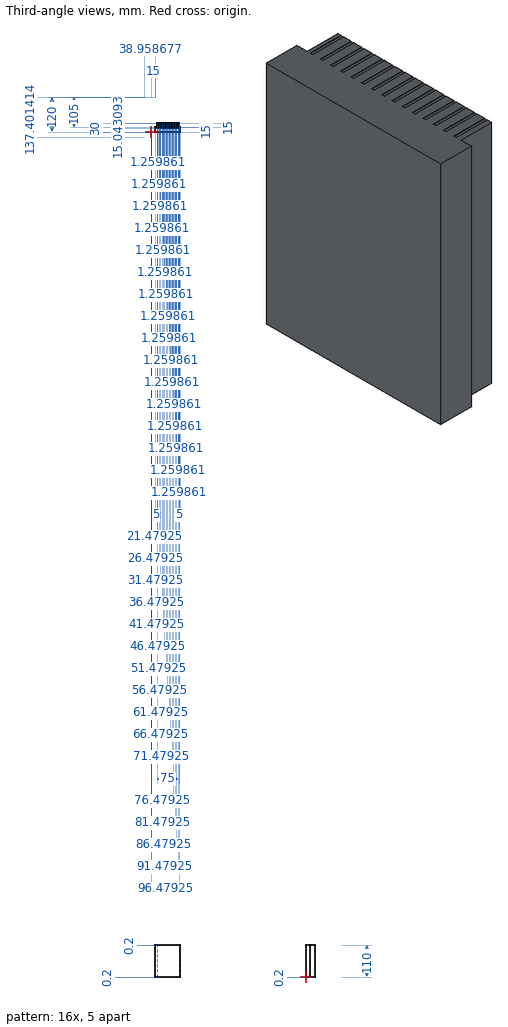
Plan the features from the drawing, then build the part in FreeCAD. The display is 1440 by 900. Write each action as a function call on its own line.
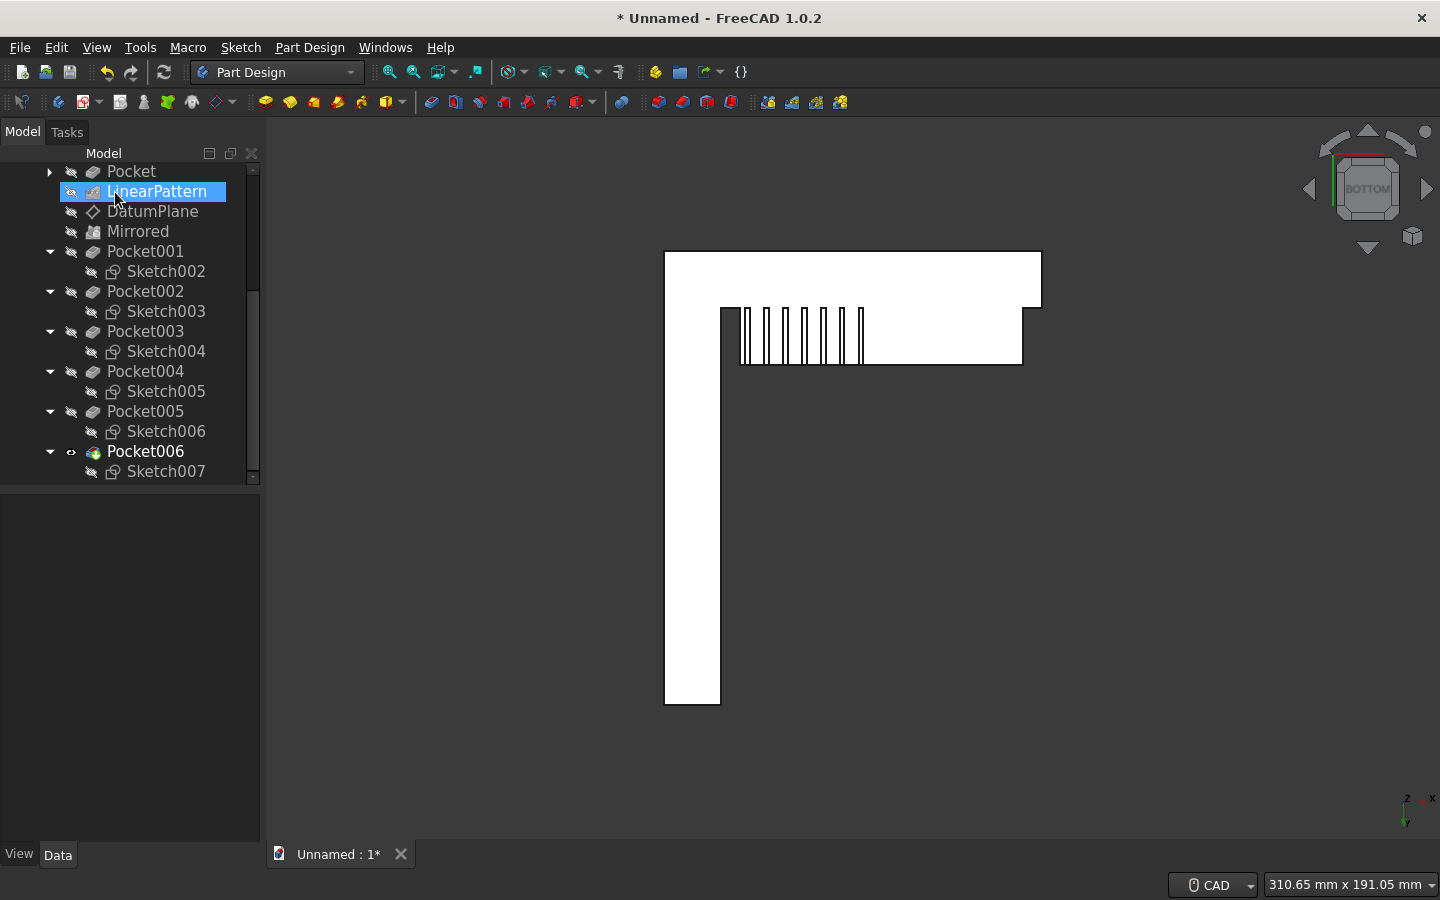
click(961, 283)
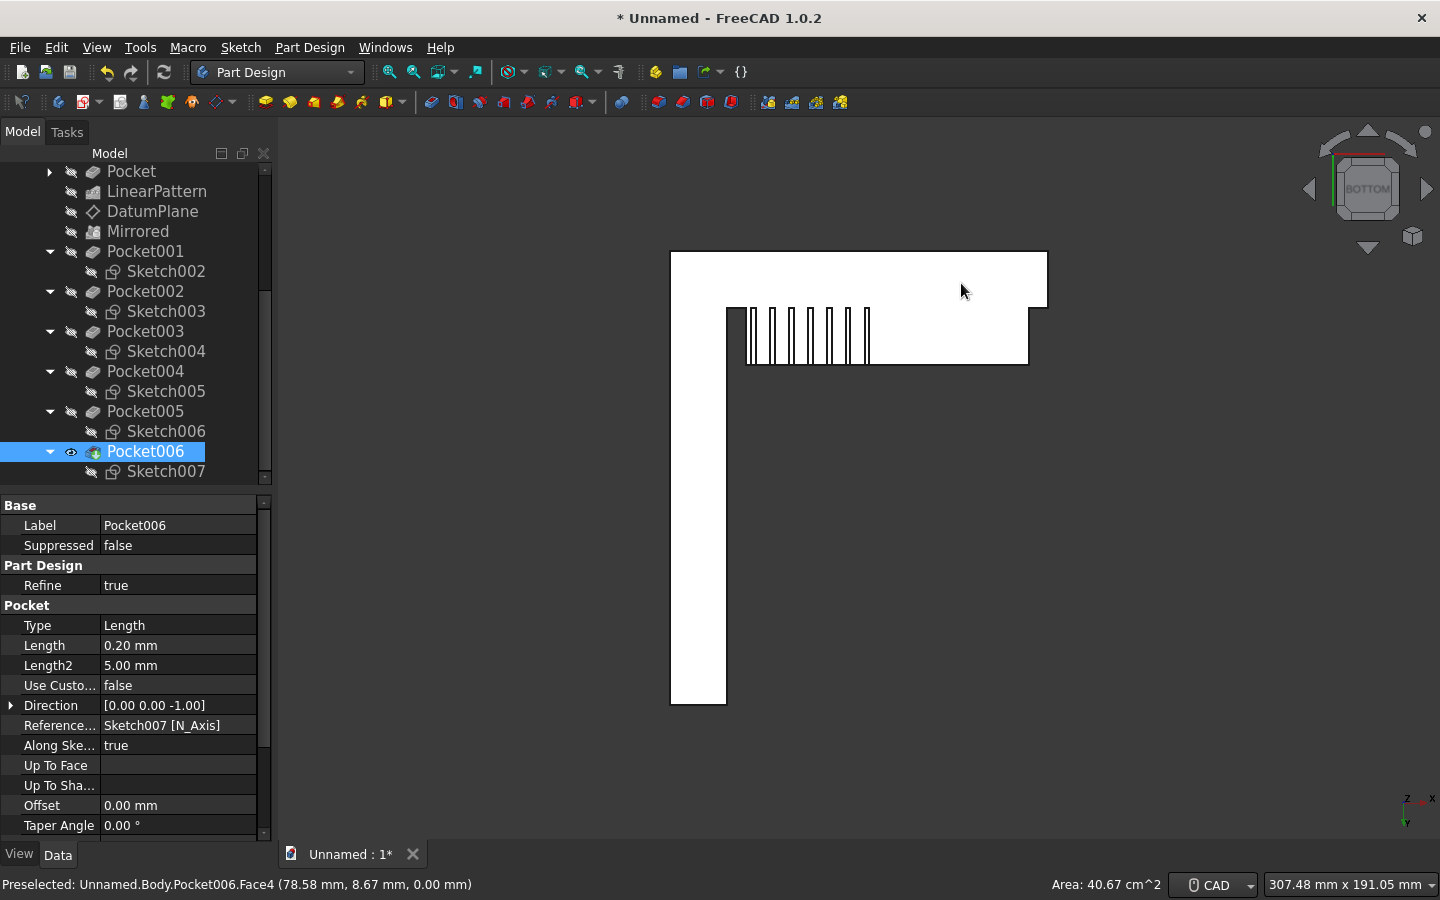
click(84, 102)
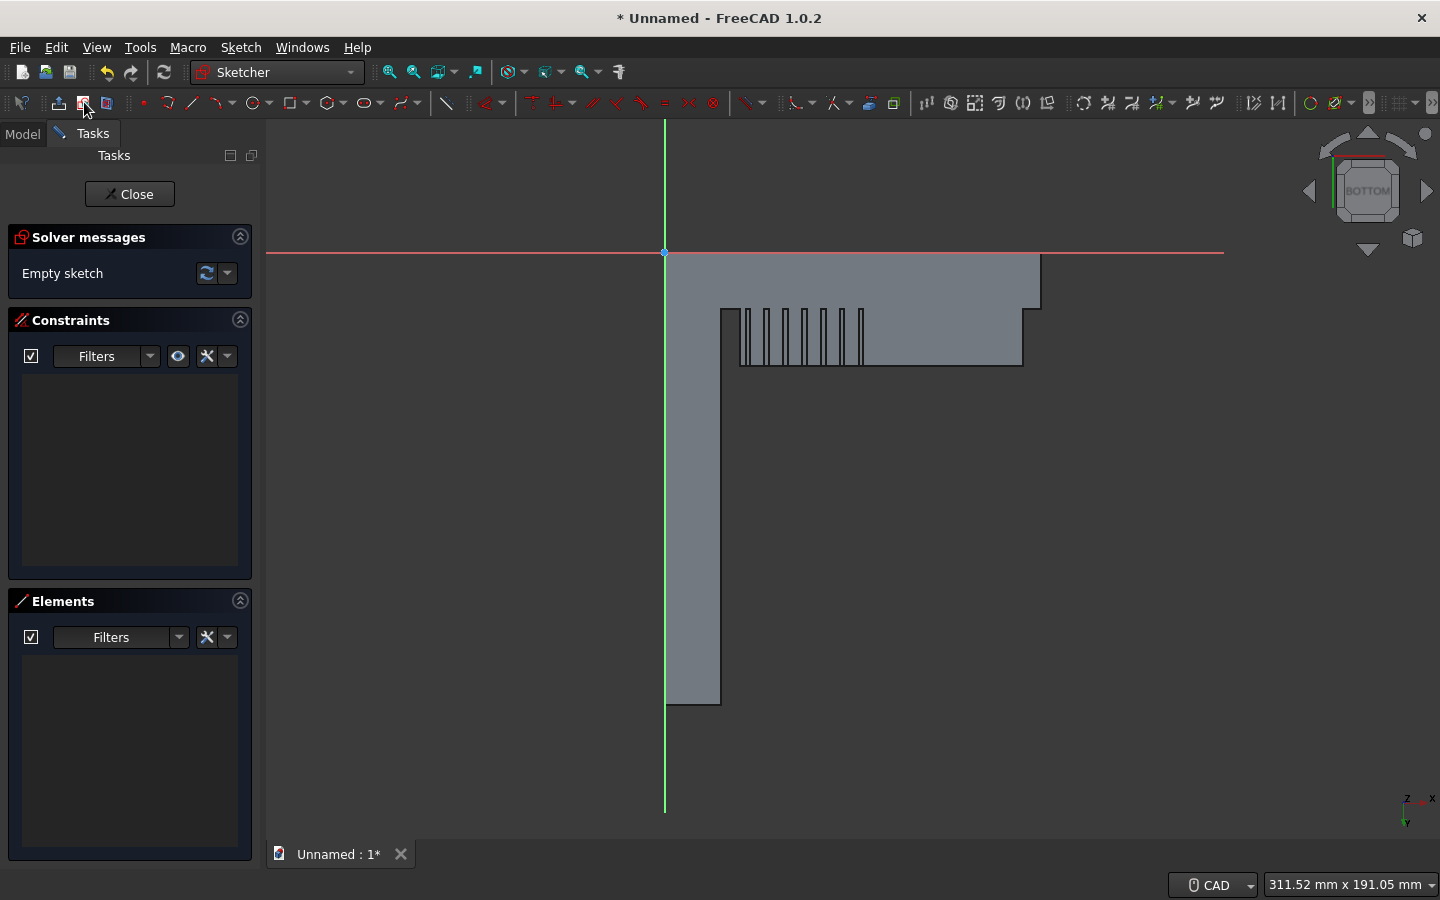
scroll(892, 320, up, 11)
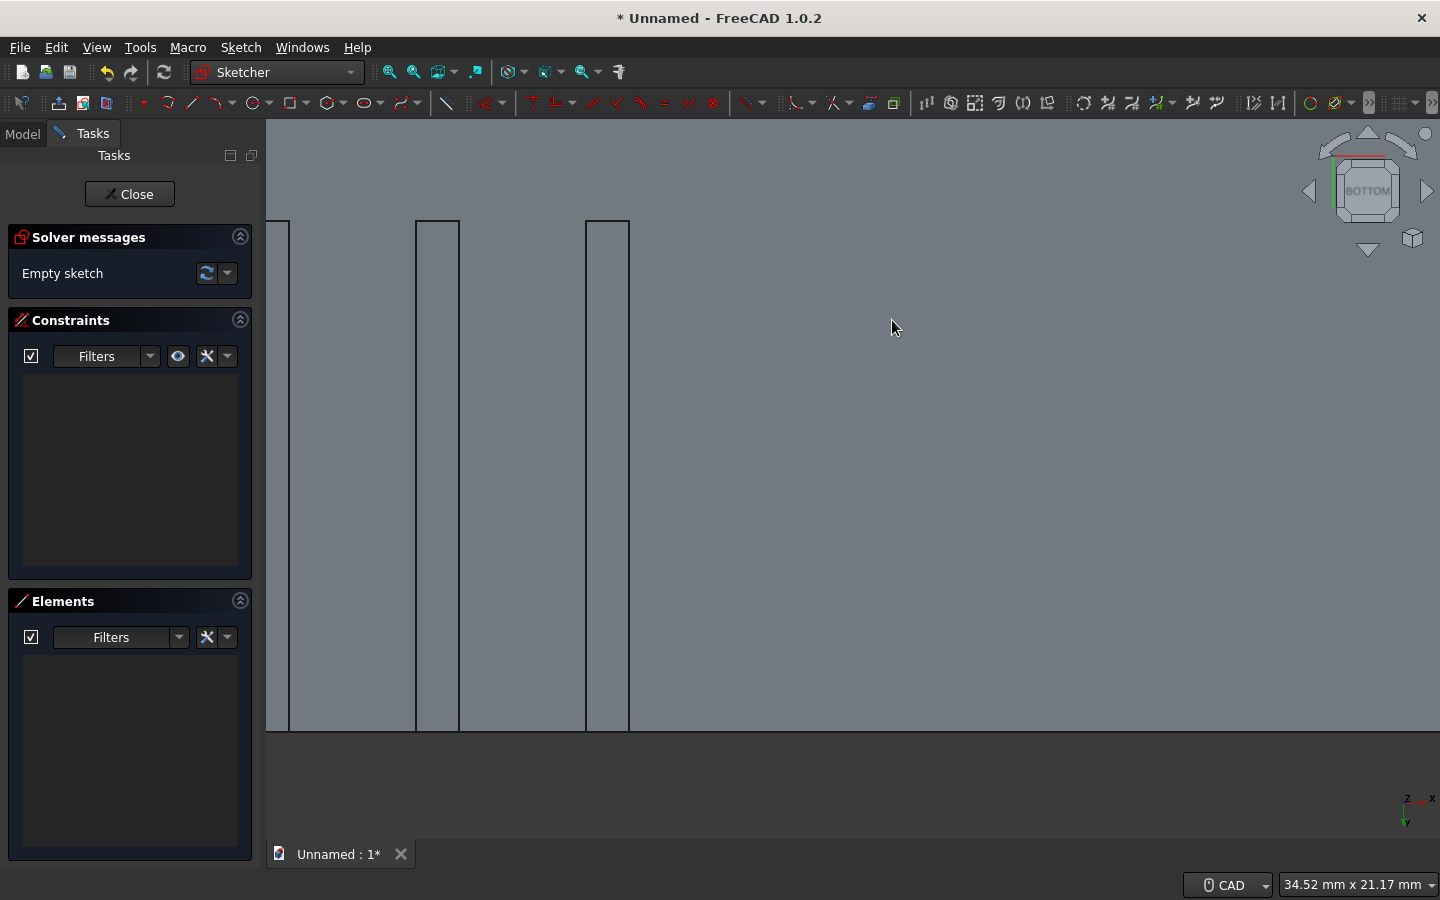
click(290, 104)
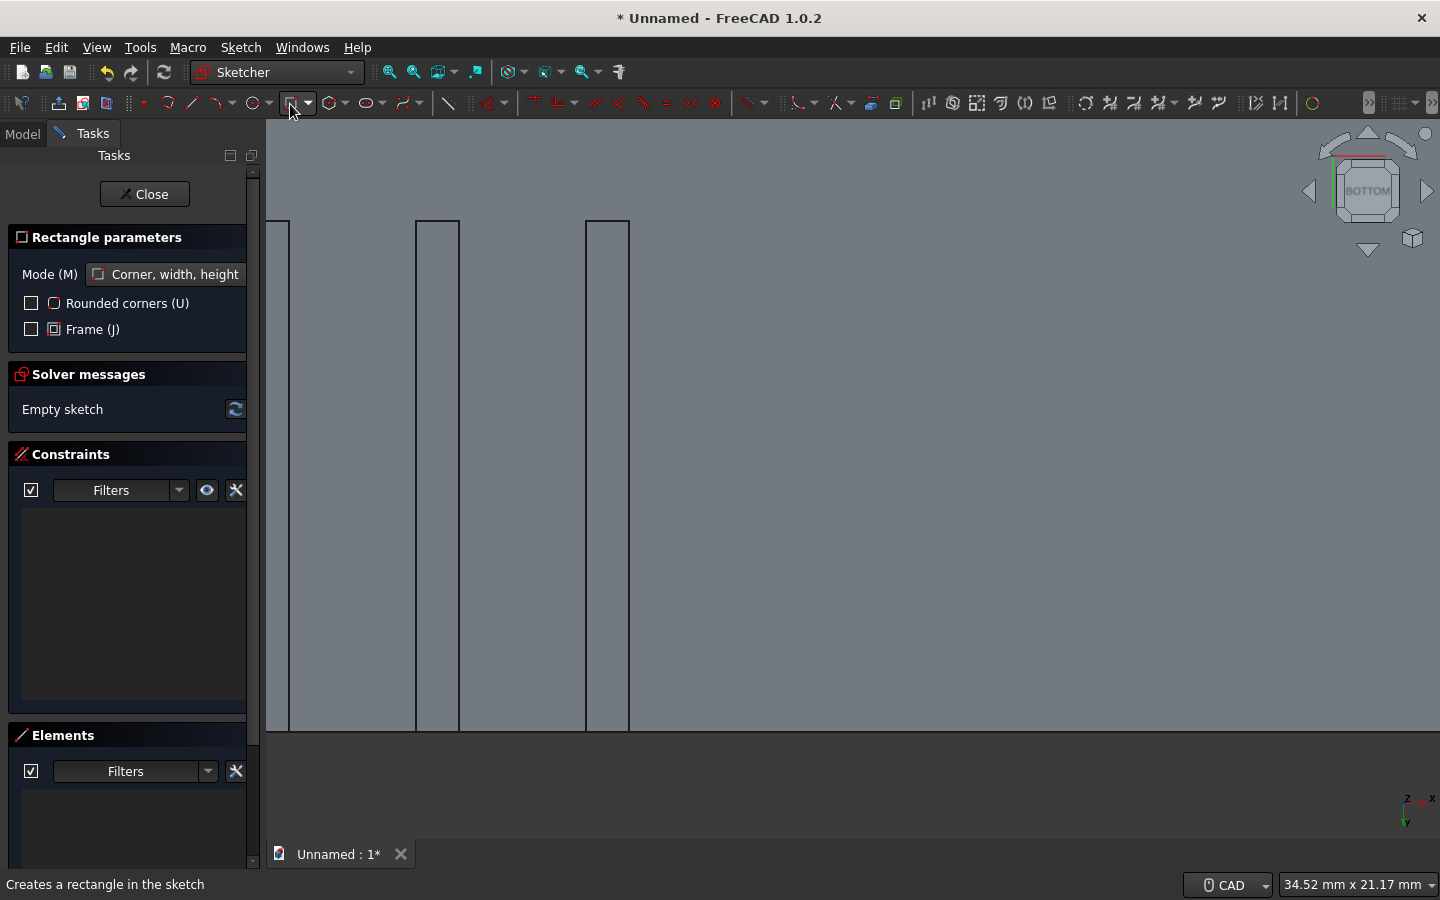
click(756, 221)
click(799, 732)
key(Escape)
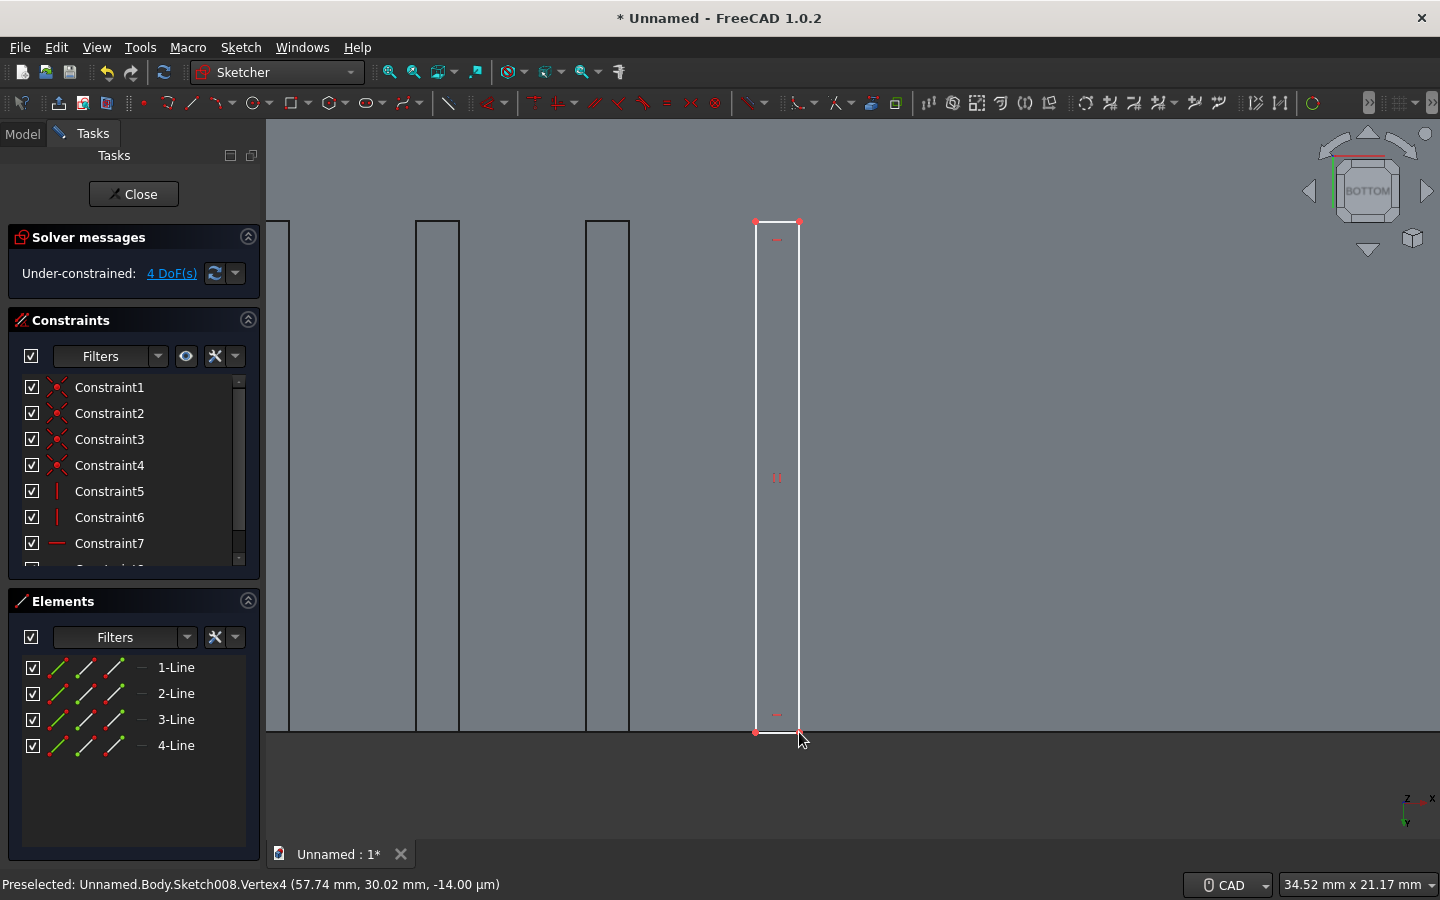
click(488, 104)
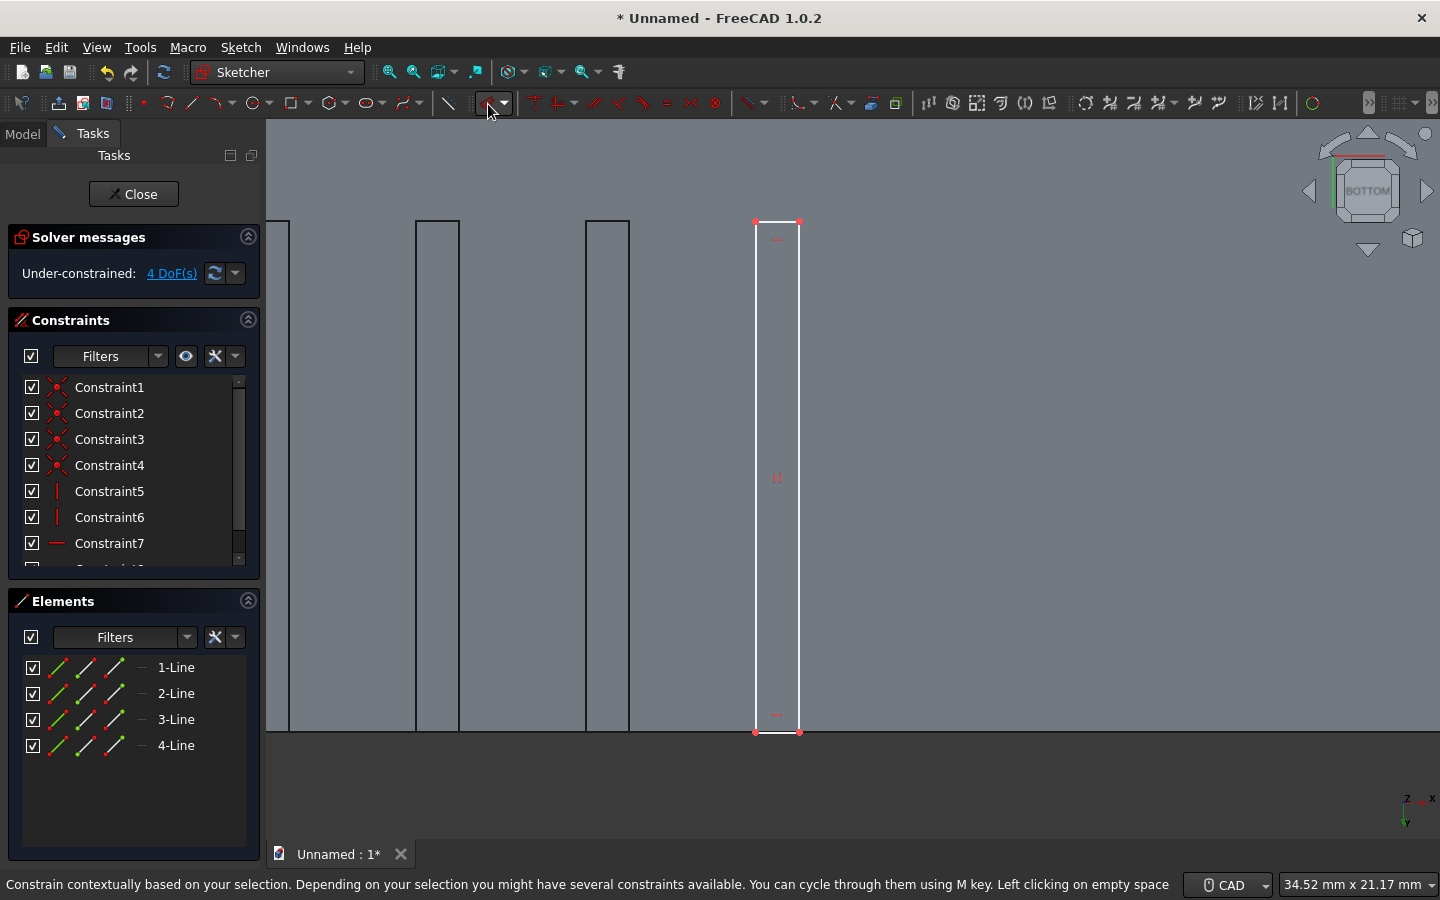
click(756, 733)
click(814, 440)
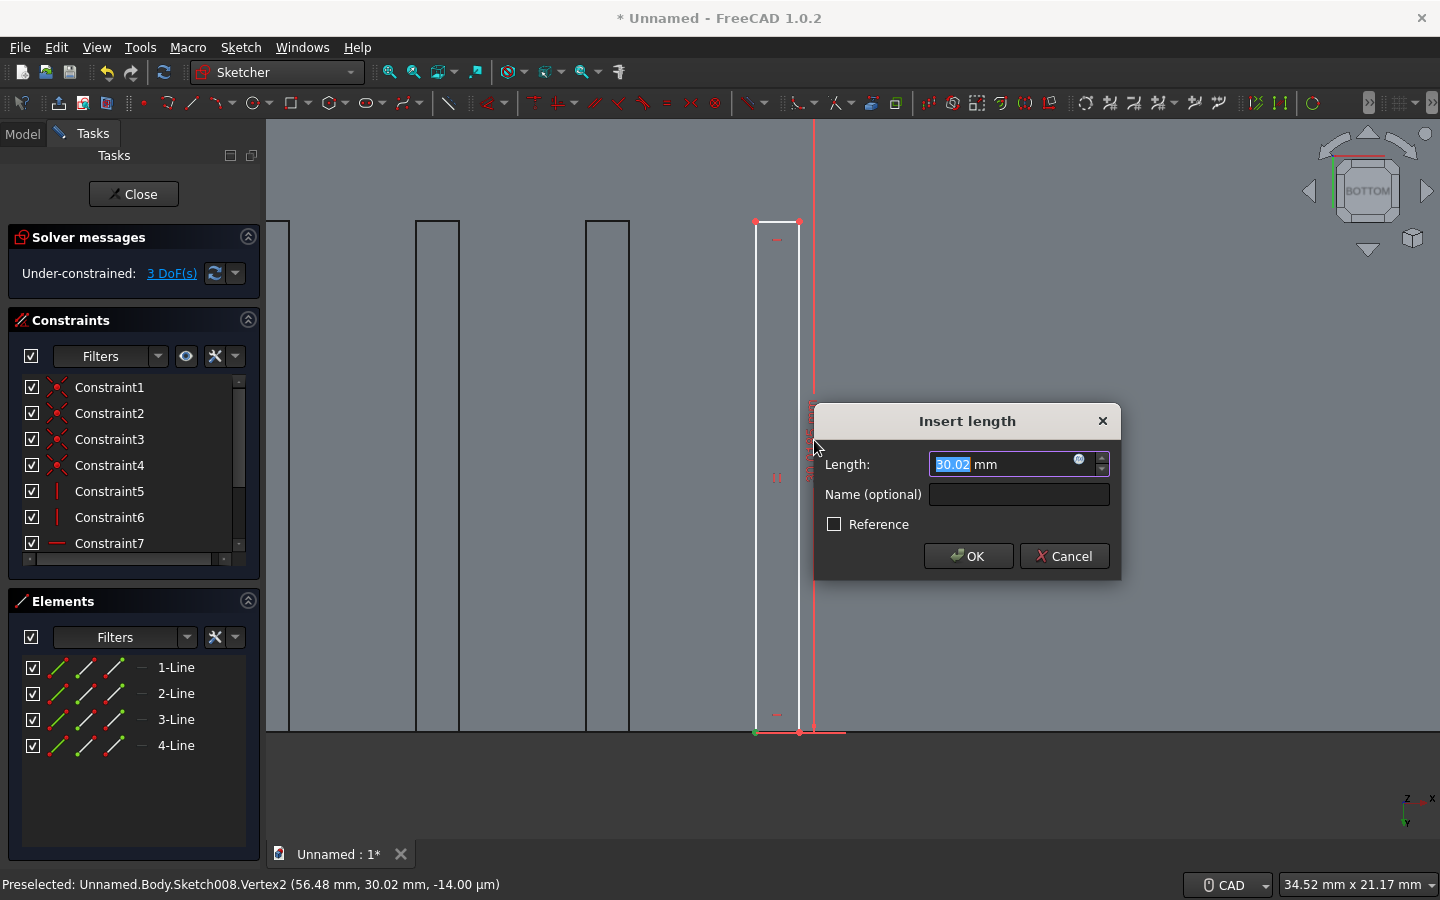
text(30)
key(Return)